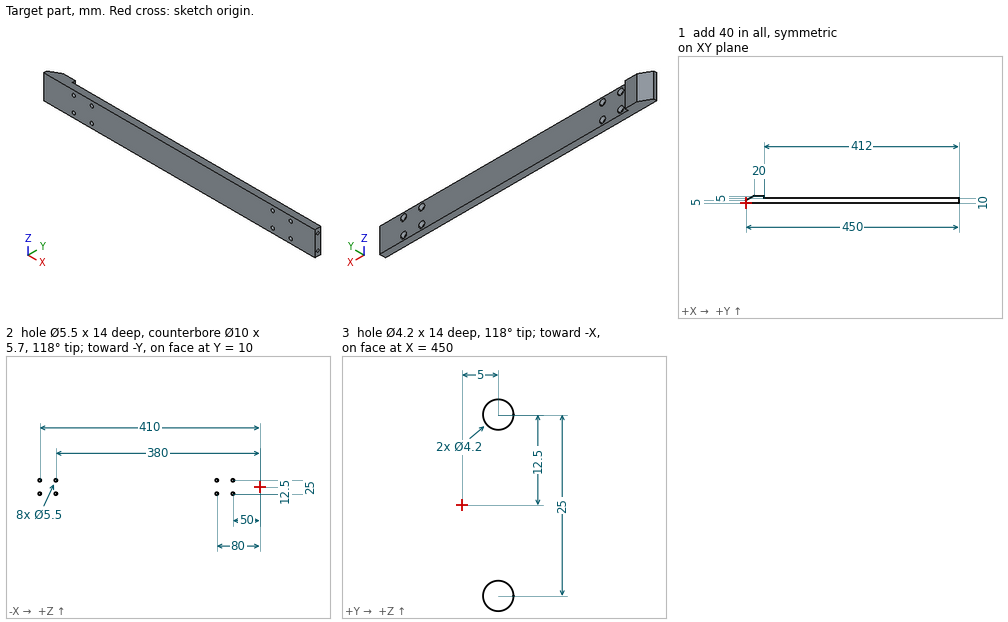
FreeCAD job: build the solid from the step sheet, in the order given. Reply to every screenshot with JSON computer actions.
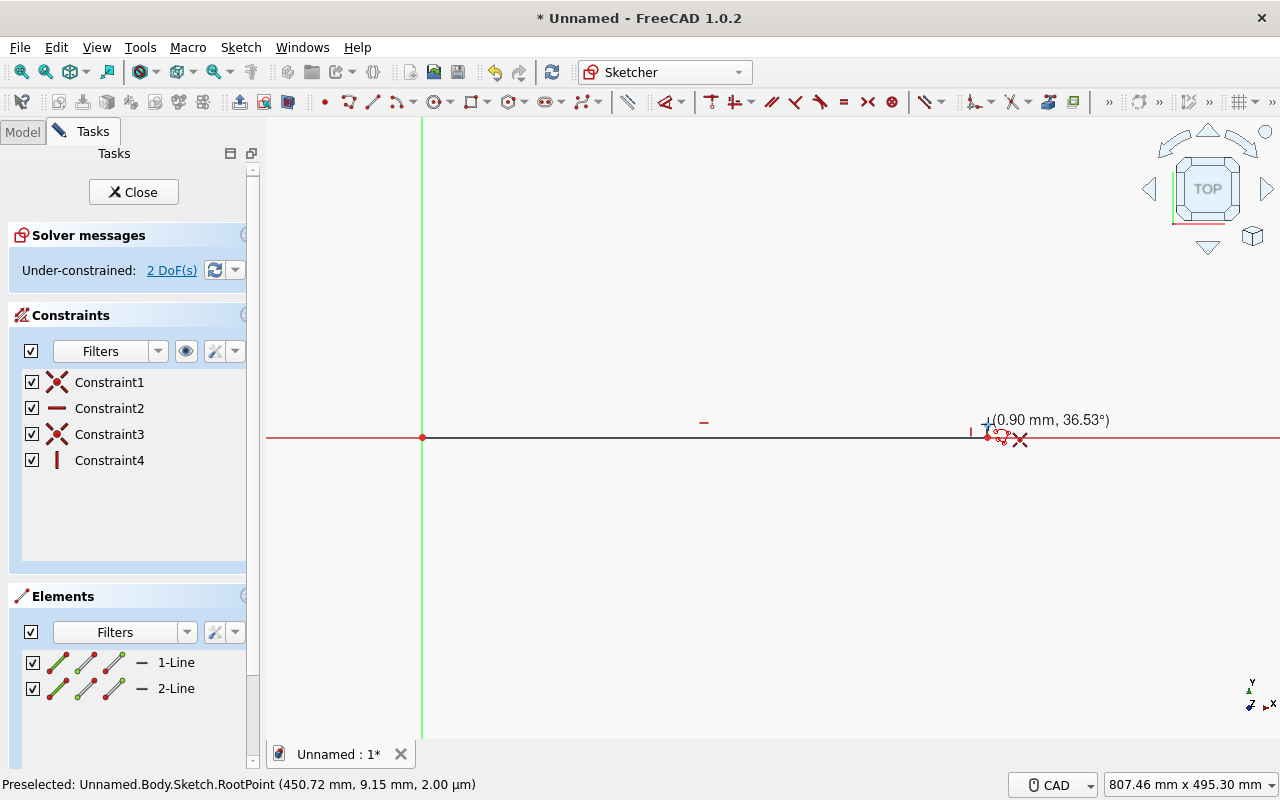
{"action": "scroll", "coordinate": [470, 425], "scroll_direction": "up", "scroll_amount": 2}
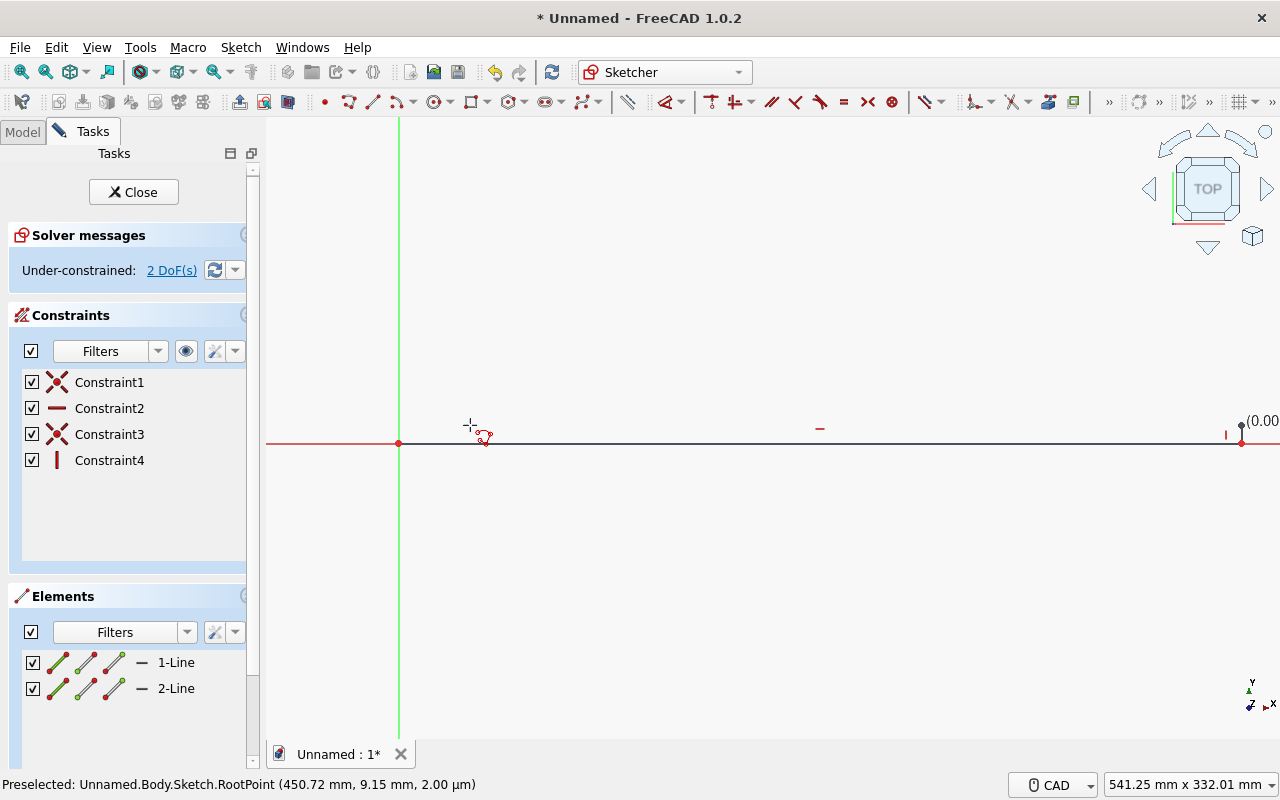
{"action": "left_click", "coordinate": [470, 425]}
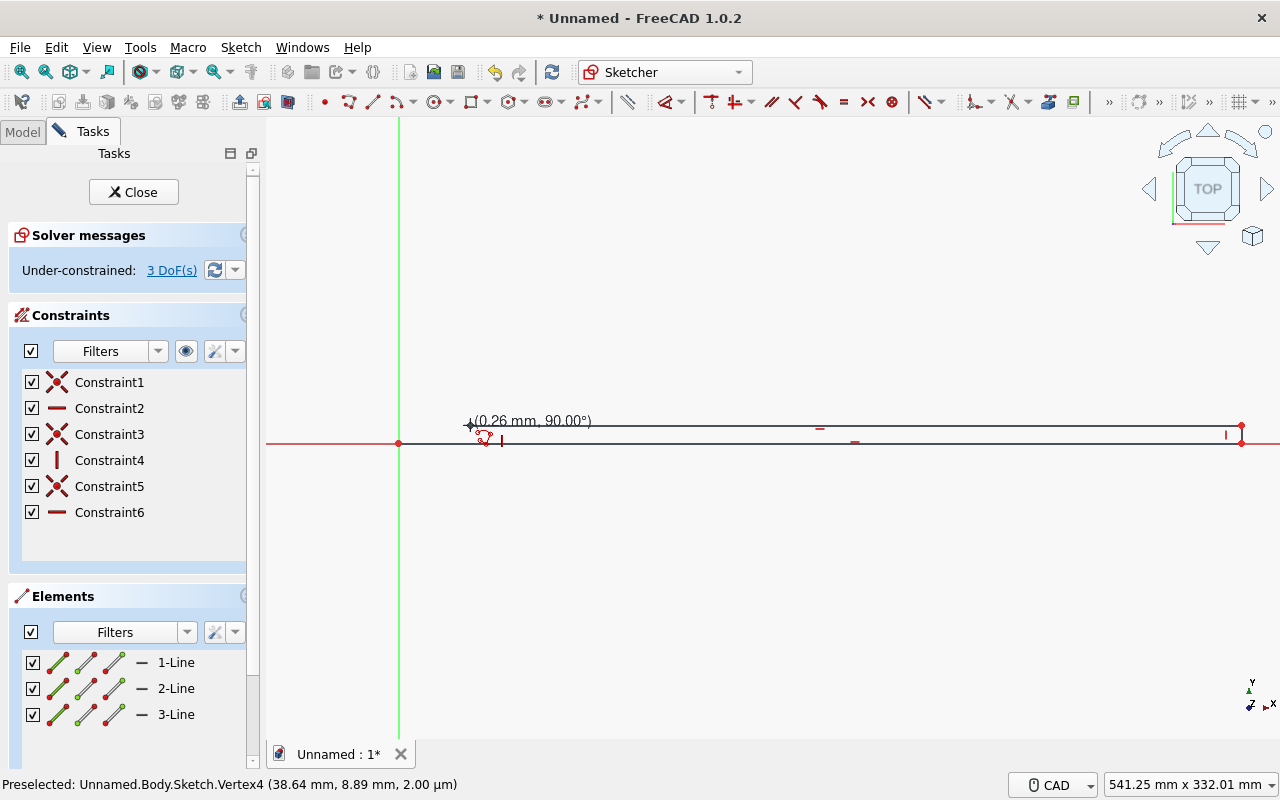
{"action": "scroll", "coordinate": [470, 416], "scroll_direction": "up", "scroll_amount": 3}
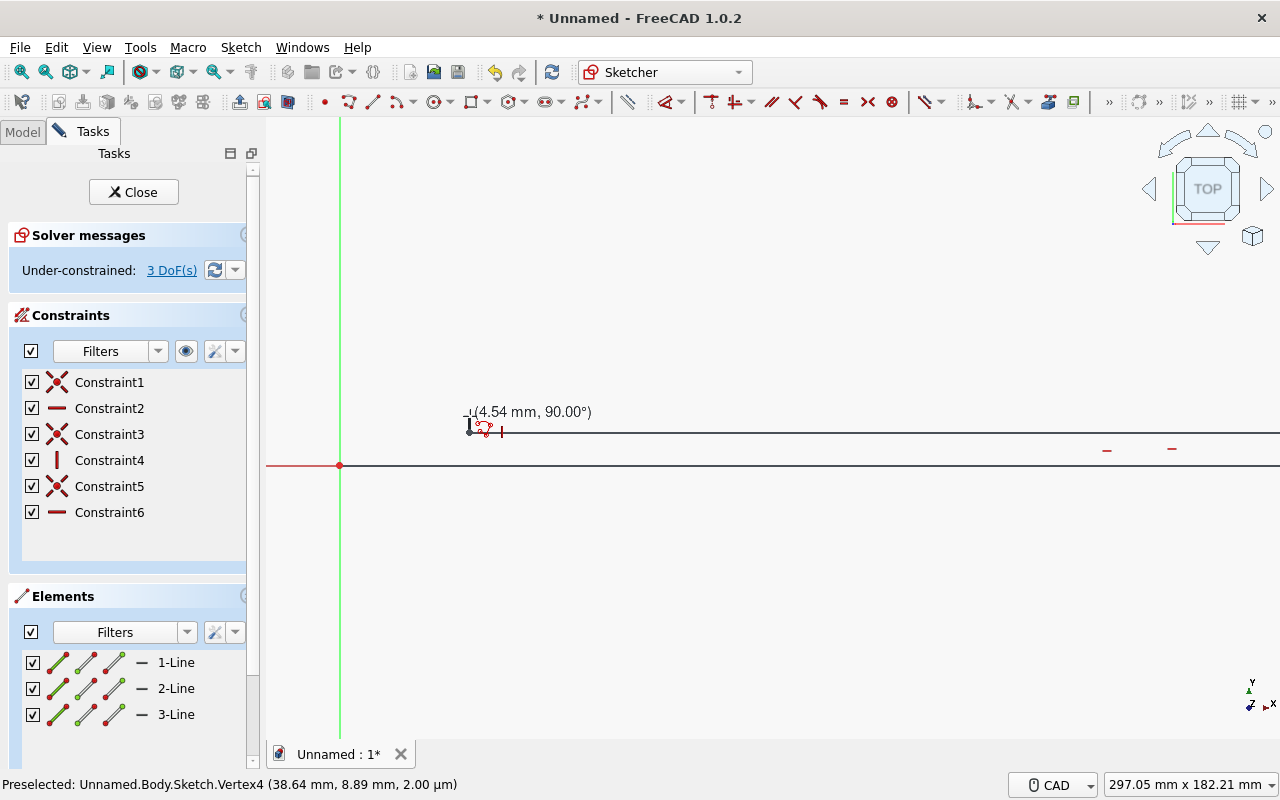
{"action": "left_click", "coordinate": [470, 415]}
{"action": "left_click", "coordinate": [401, 415]}
{"action": "left_click", "coordinate": [349, 449]}
{"action": "left_click", "coordinate": [340, 466]}
{"action": "key", "text": "Escape"}
{"action": "key", "text": "Escape"}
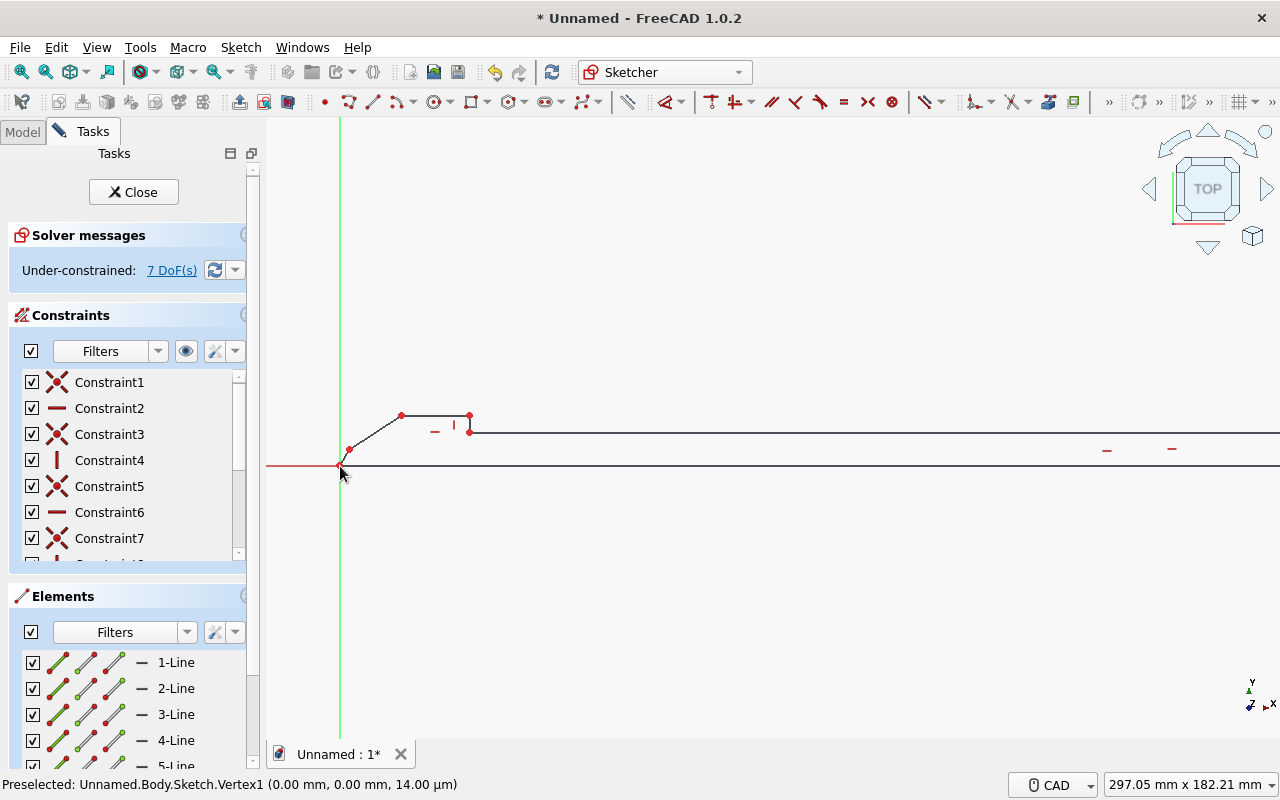
{"action": "scroll", "coordinate": [343, 460], "scroll_direction": "up", "scroll_amount": 4}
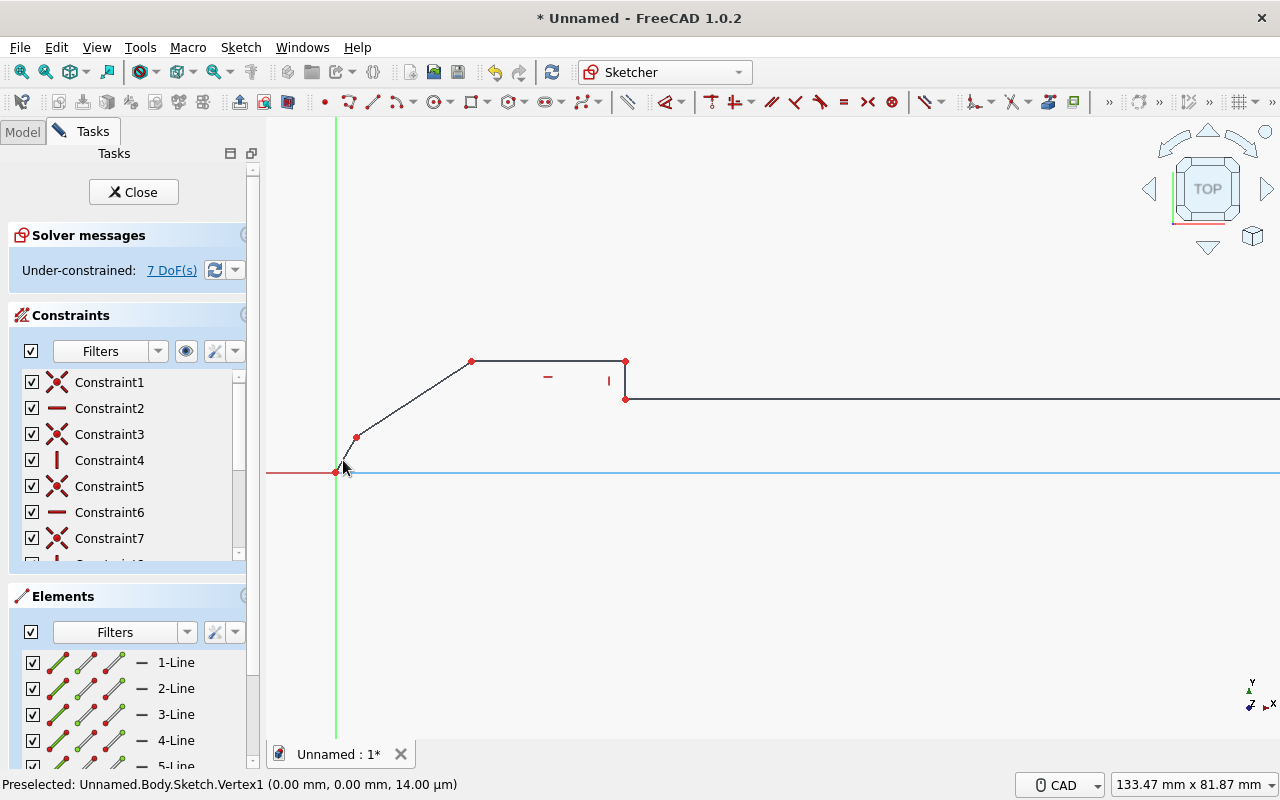
{"action": "left_click", "coordinate": [344, 458]}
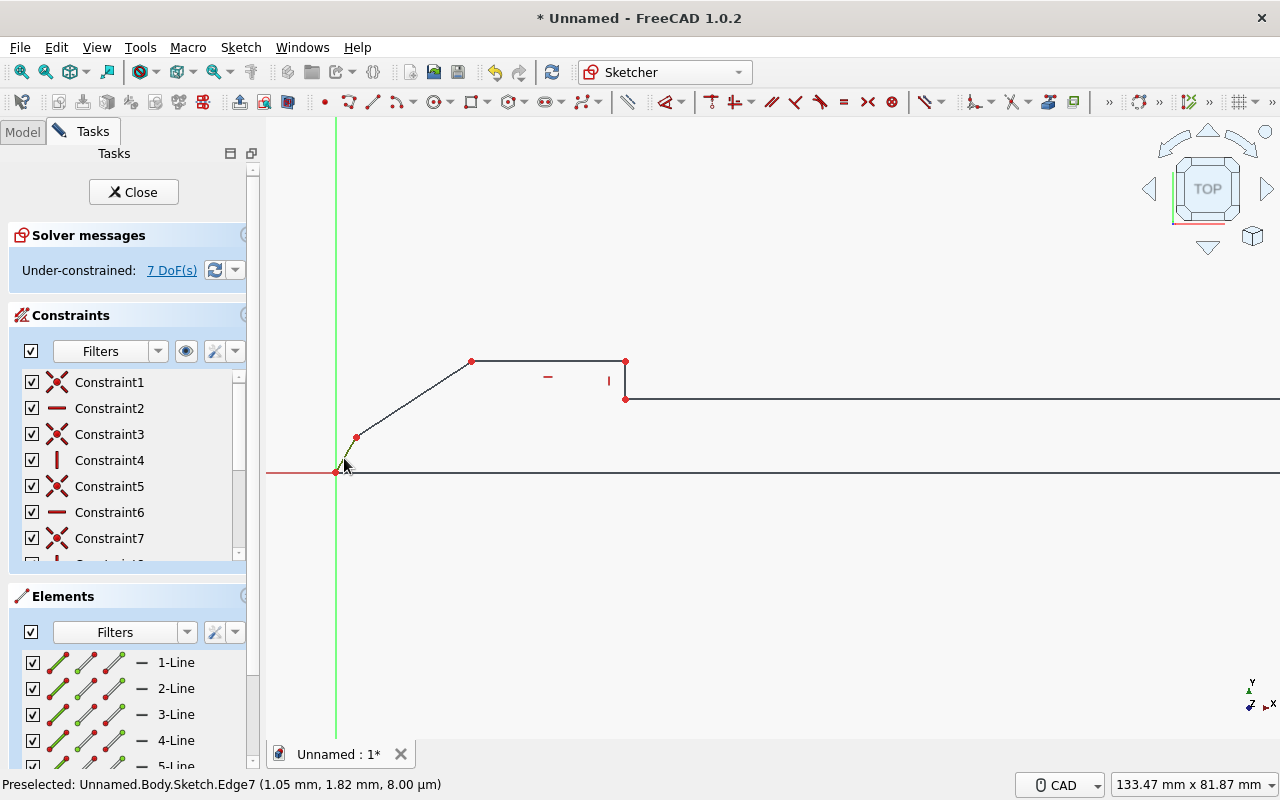
{"action": "left_click", "coordinate": [754, 102]}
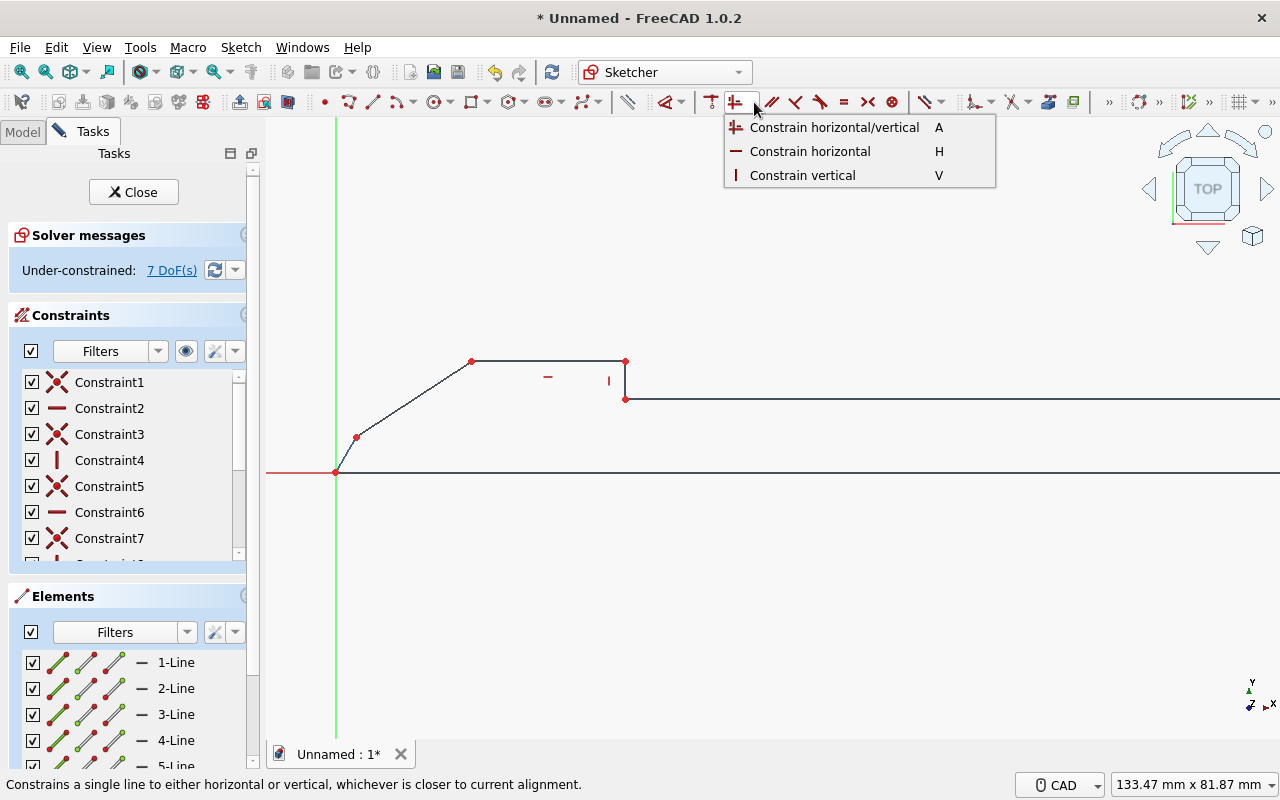
{"action": "left_click", "coordinate": [860, 175]}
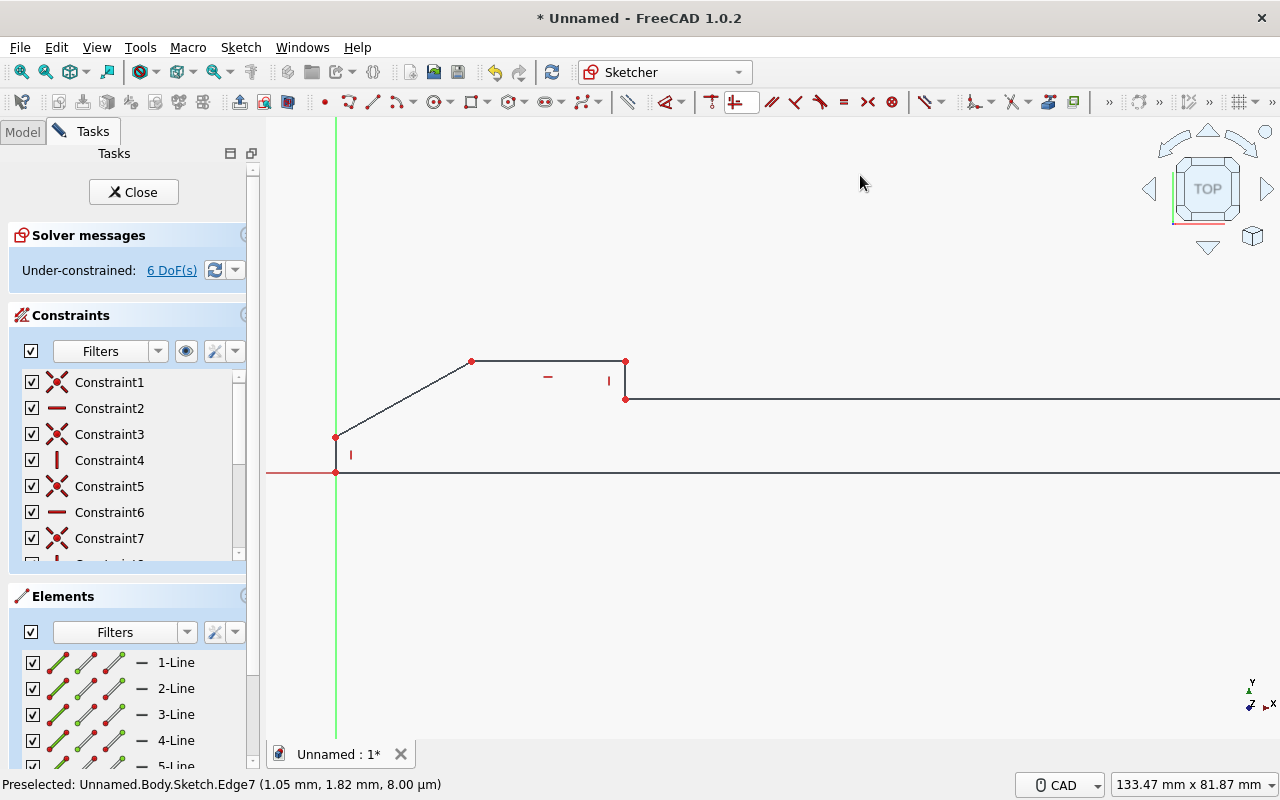
{"action": "scroll", "coordinate": [625, 388], "scroll_direction": "up", "scroll_amount": 2}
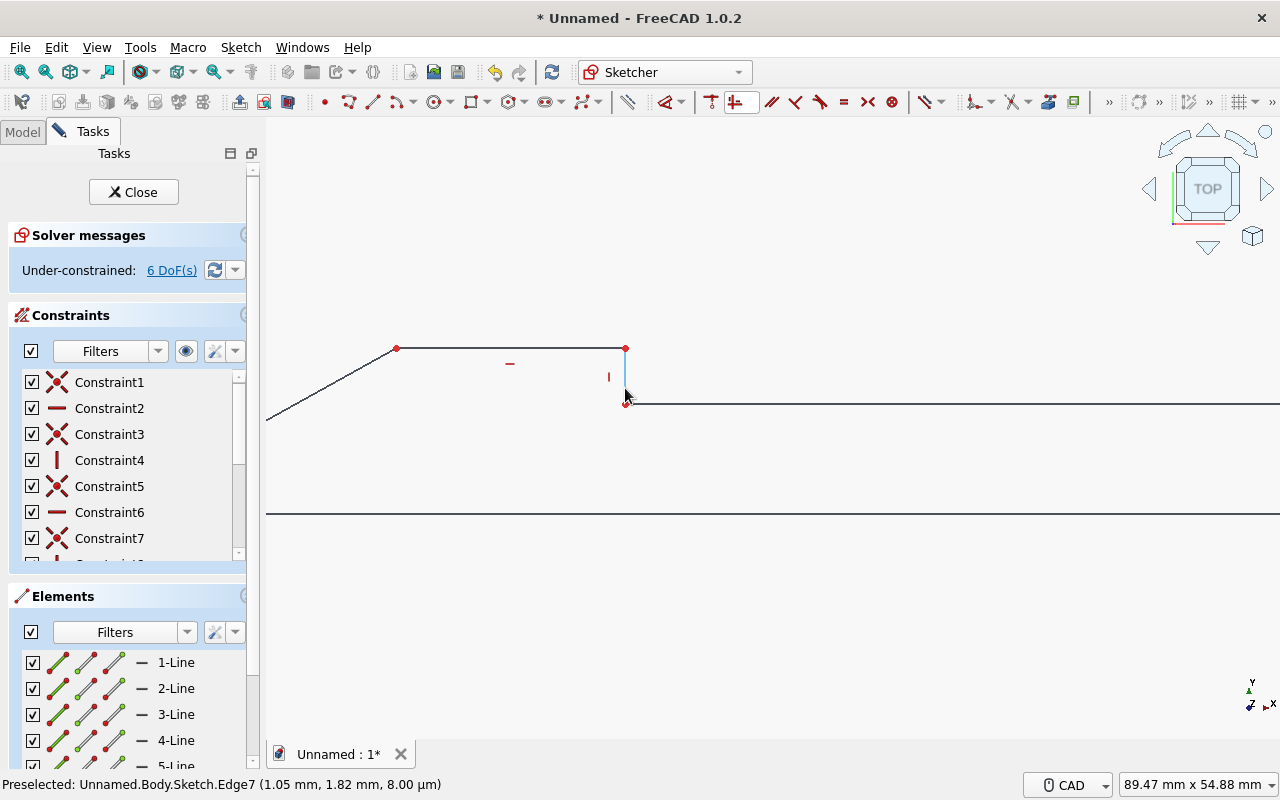
{"action": "left_click", "coordinate": [625, 387]}